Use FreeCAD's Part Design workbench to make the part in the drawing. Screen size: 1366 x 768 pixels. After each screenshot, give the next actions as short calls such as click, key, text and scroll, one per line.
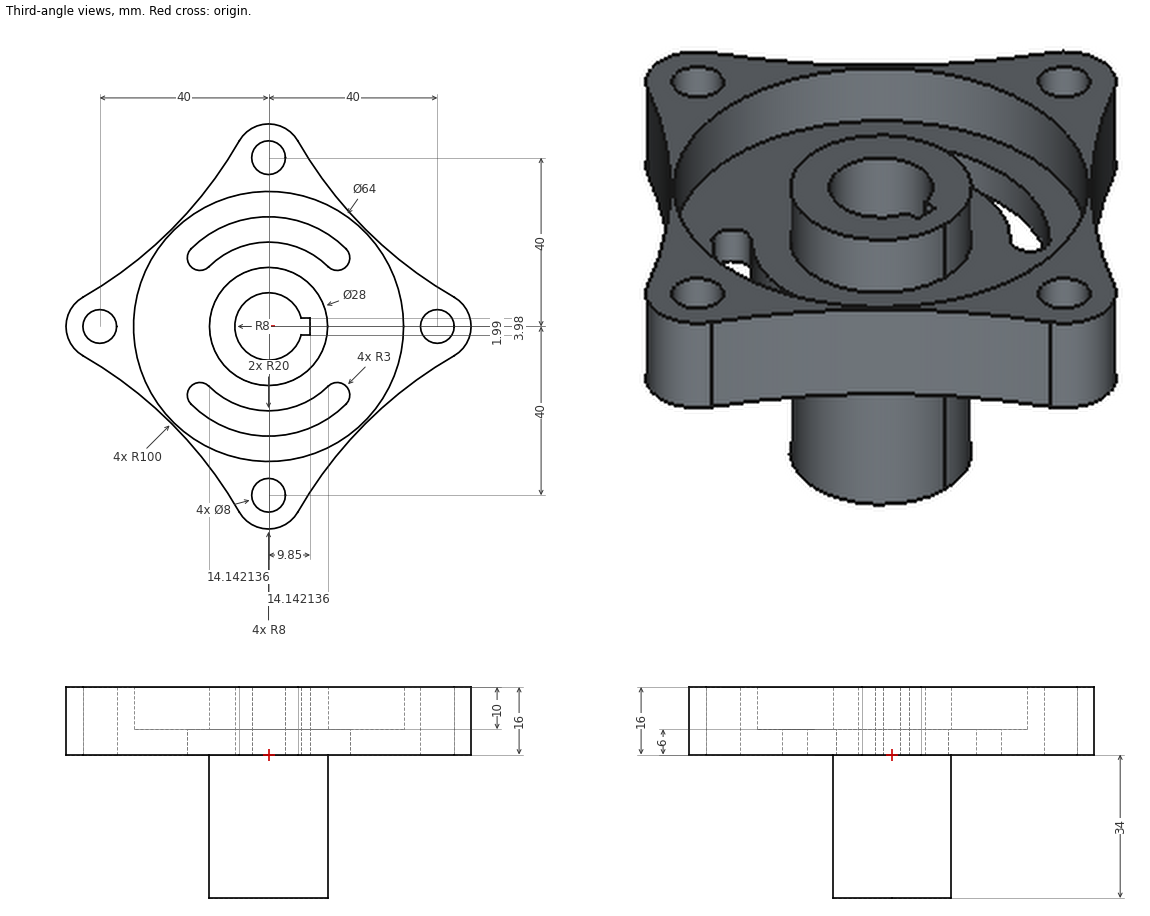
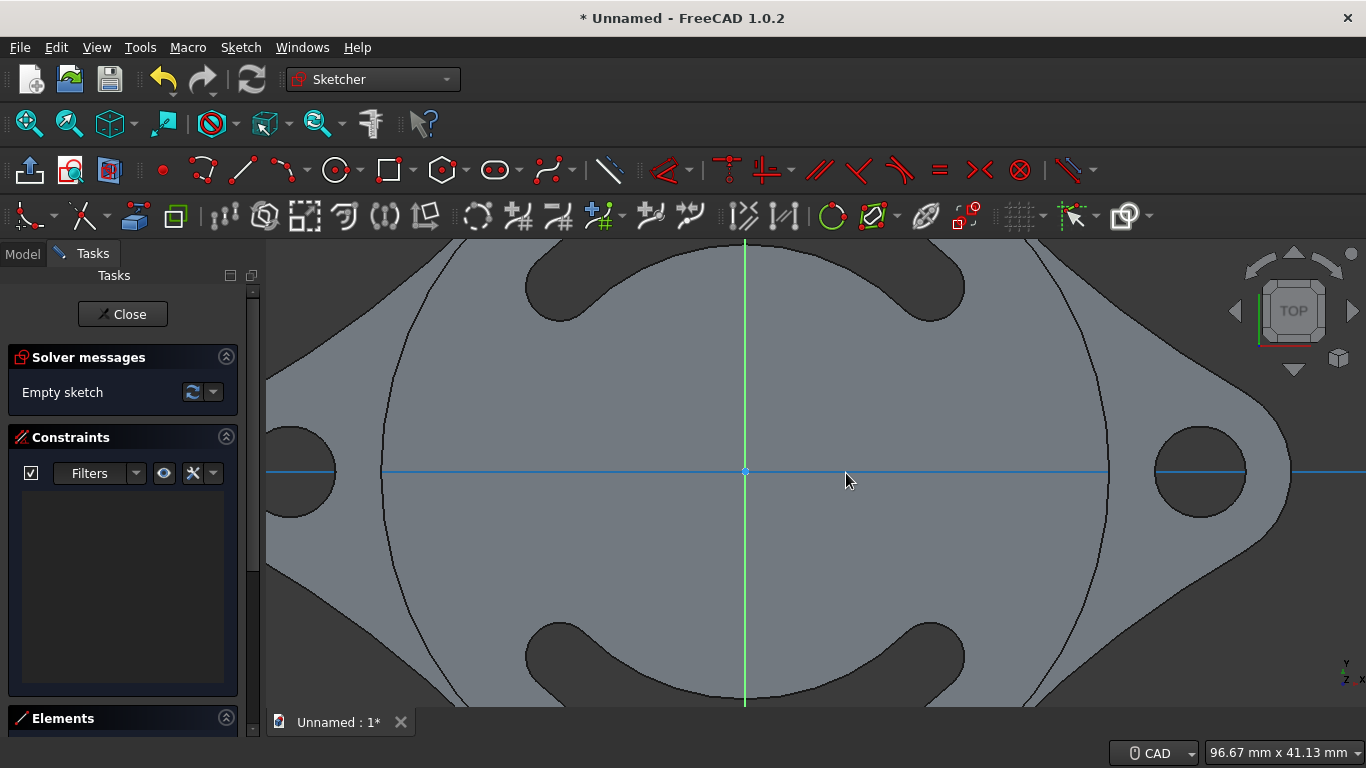
click(336, 170)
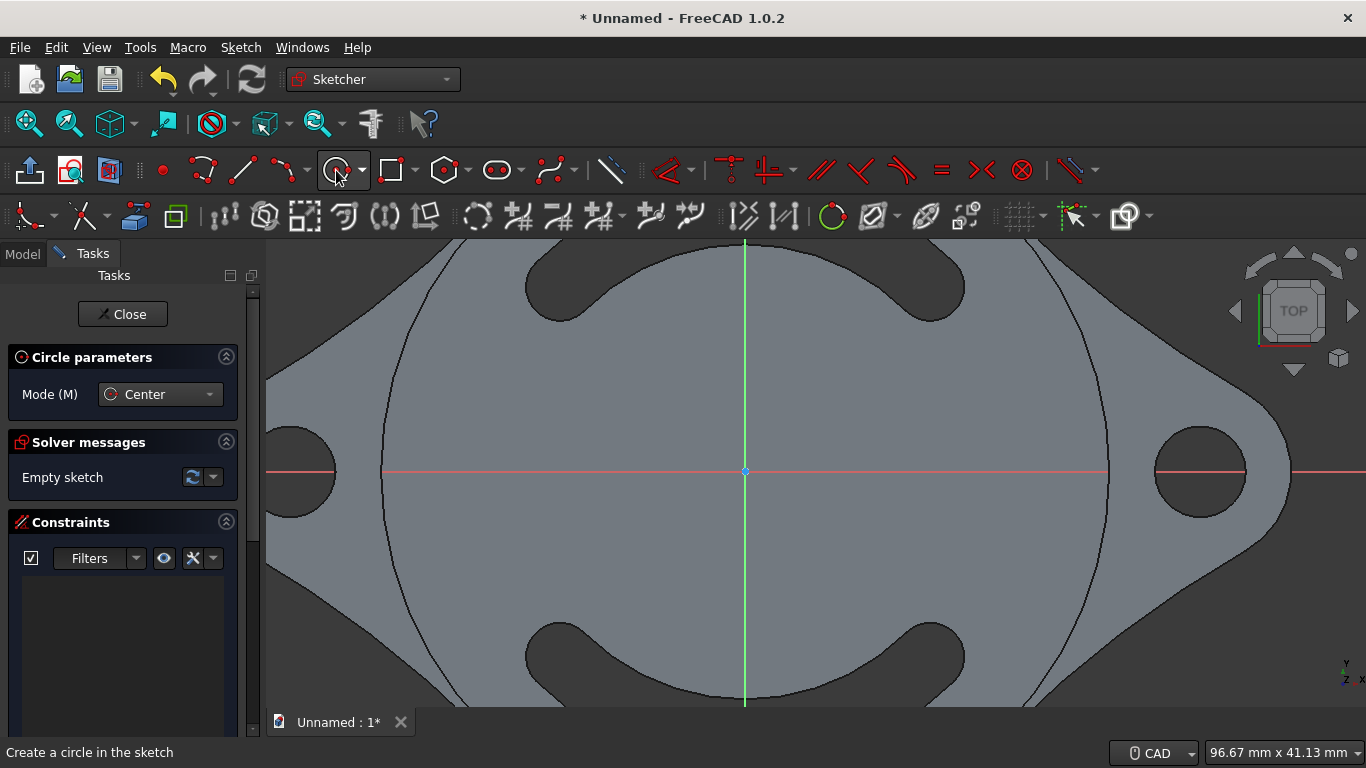
click(745, 472)
move(858, 359)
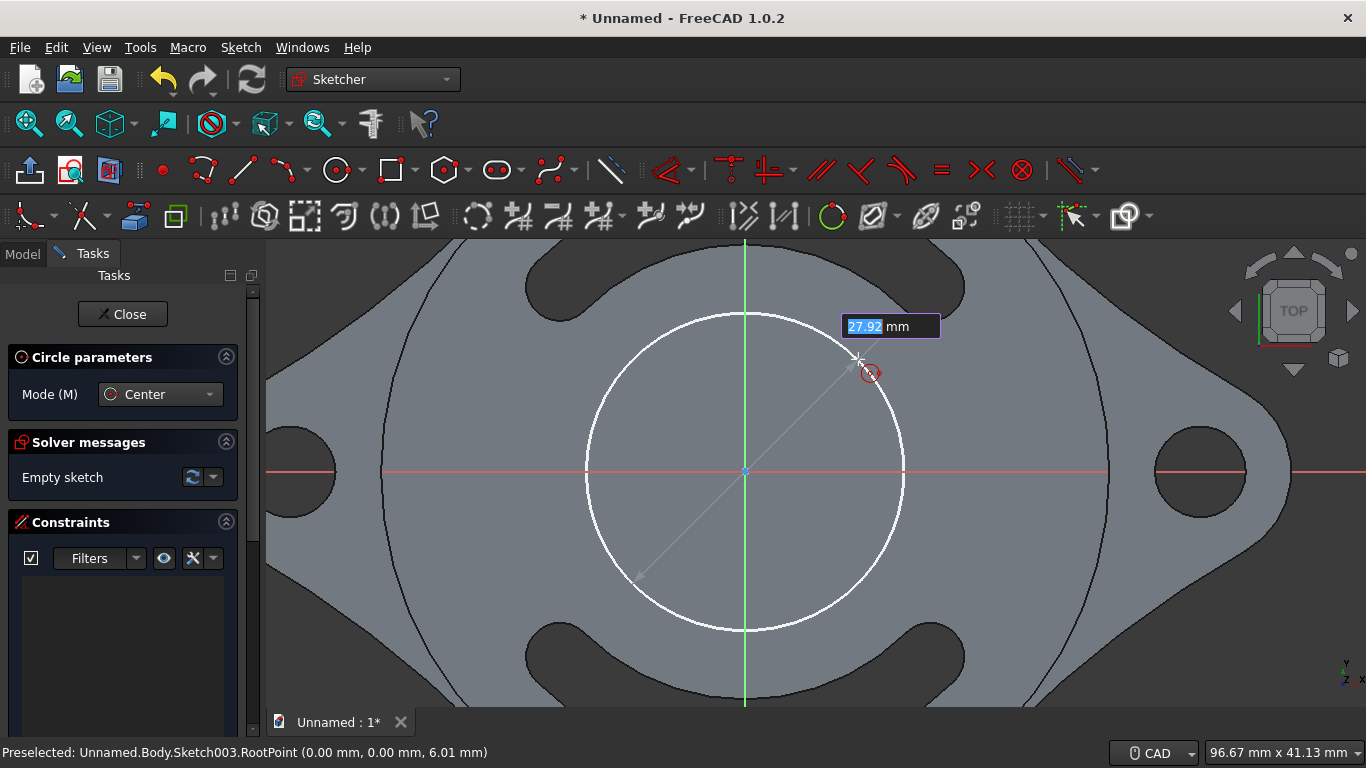
text(28)
key(Return)
key(Escape)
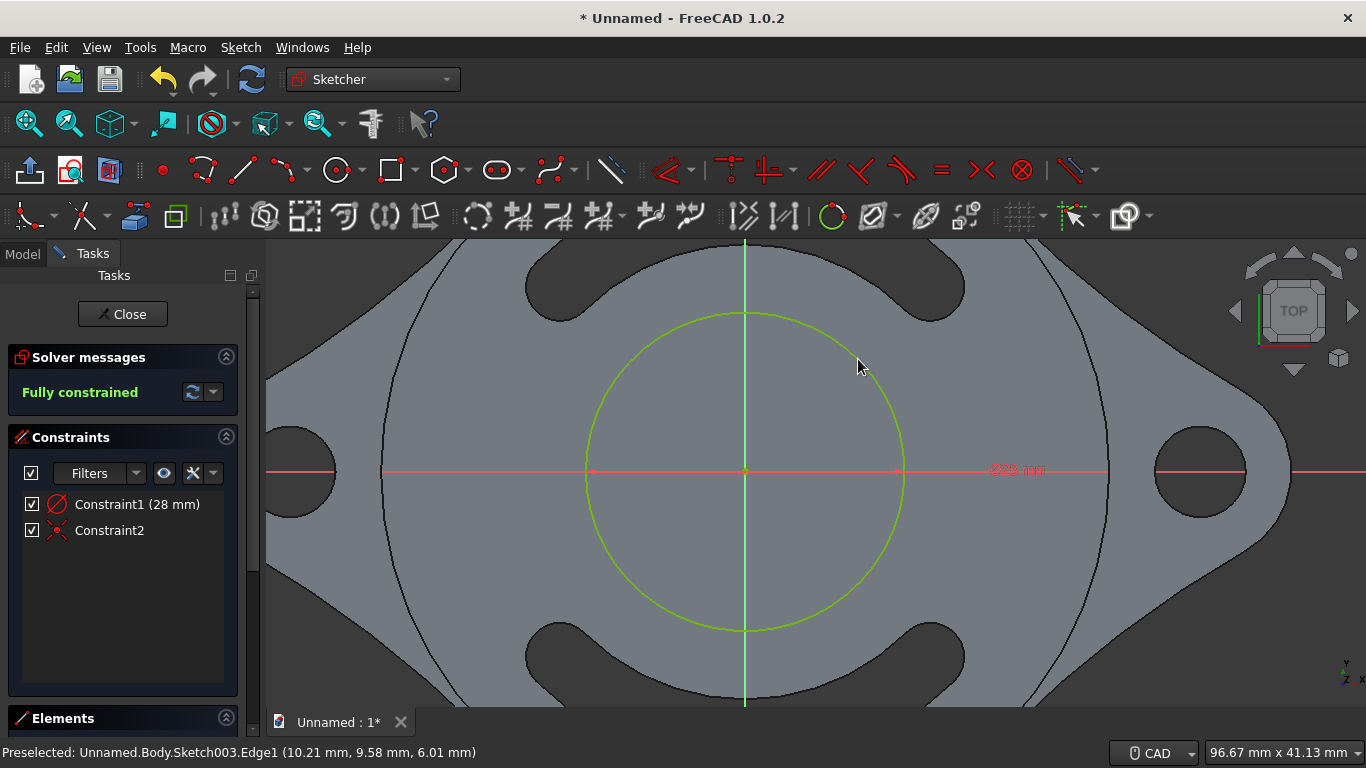
click(123, 314)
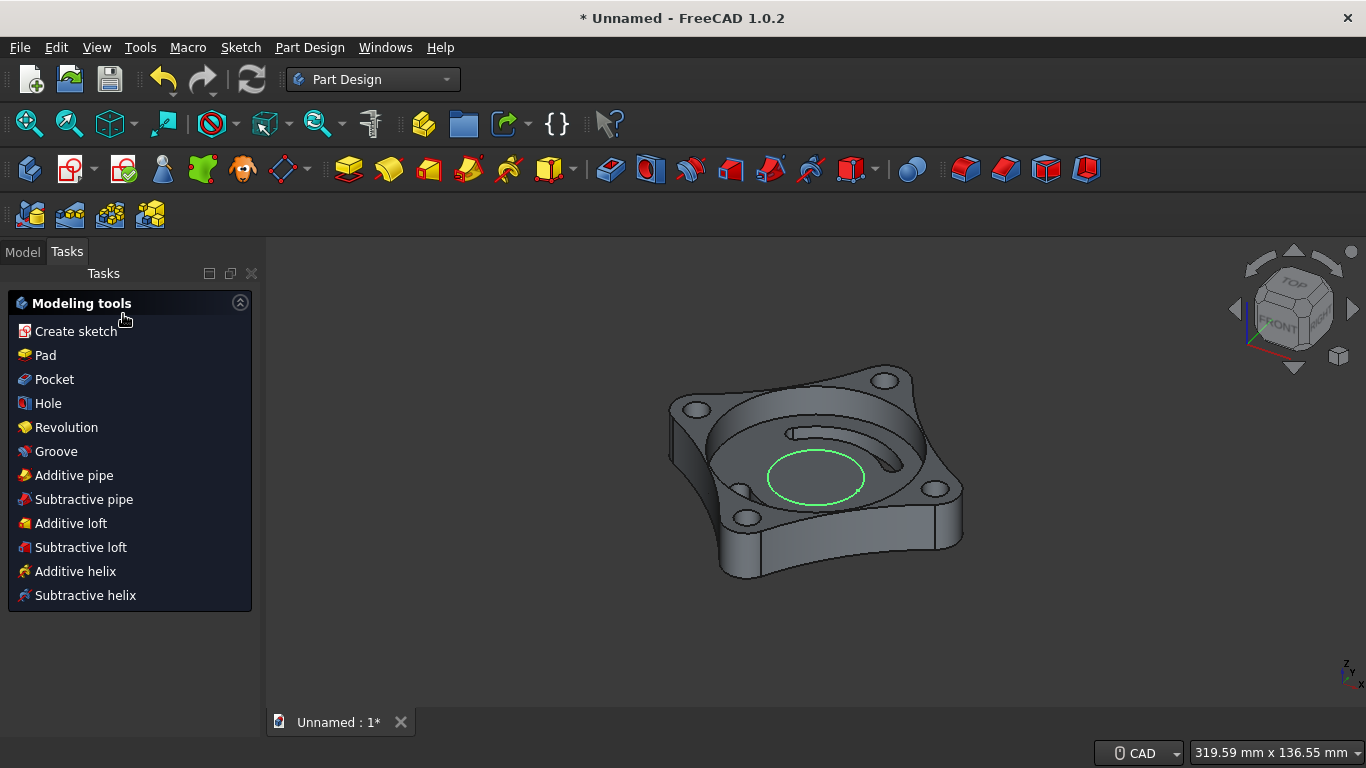
click(350, 170)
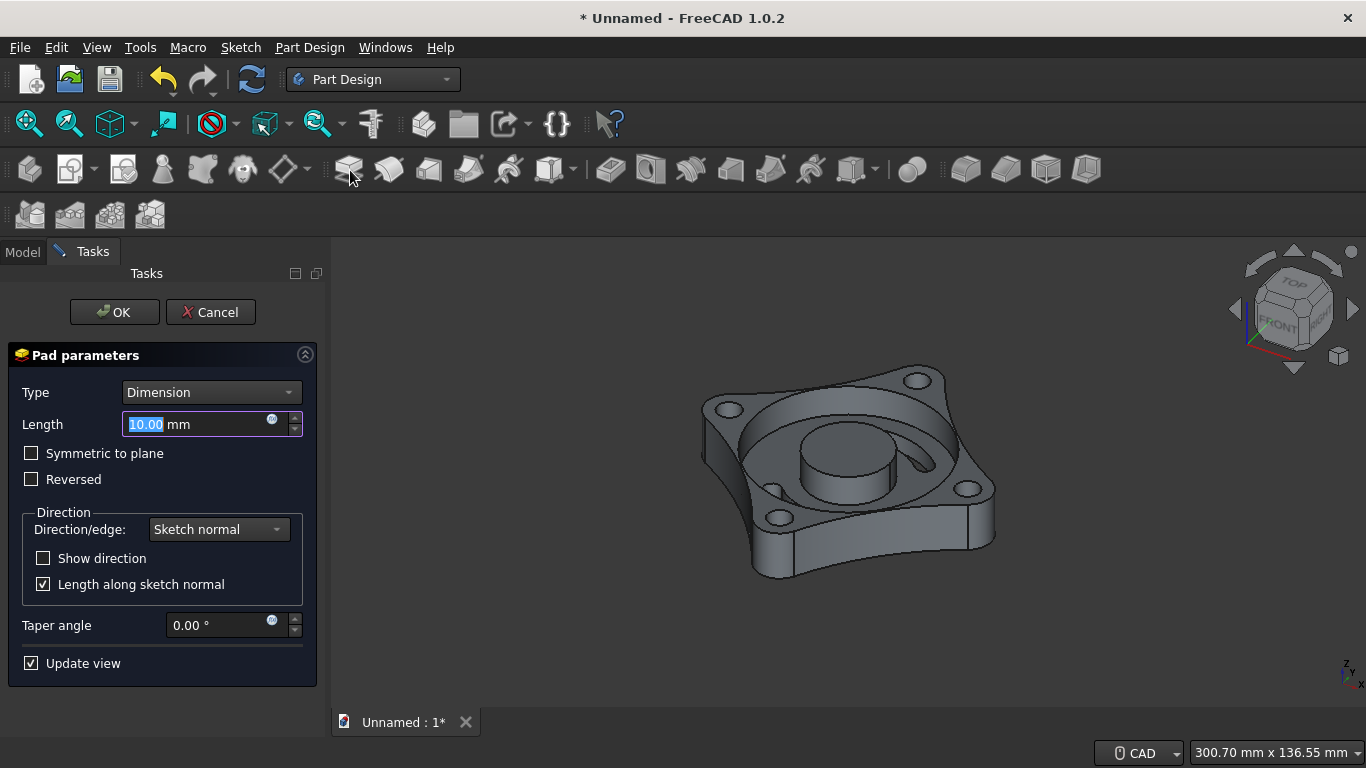
text(10)
key(Tab)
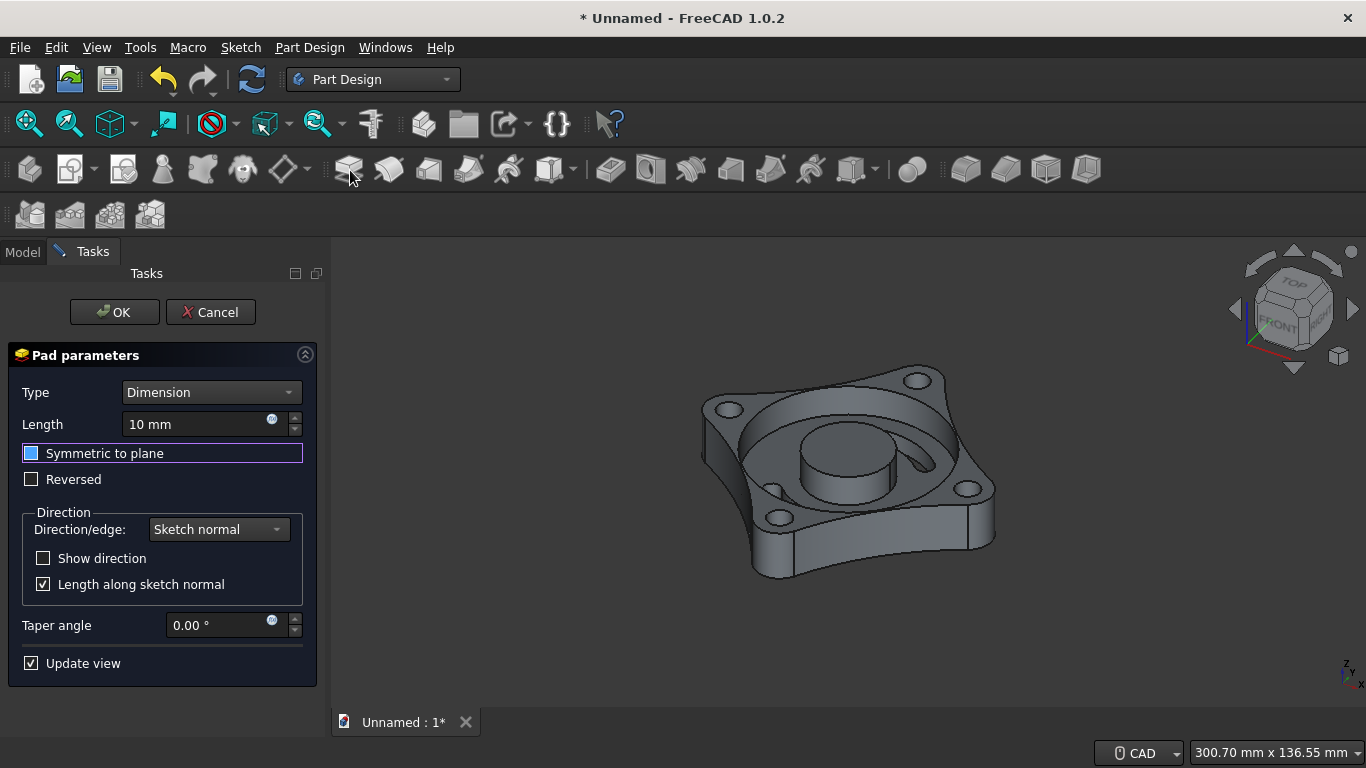
click(115, 312)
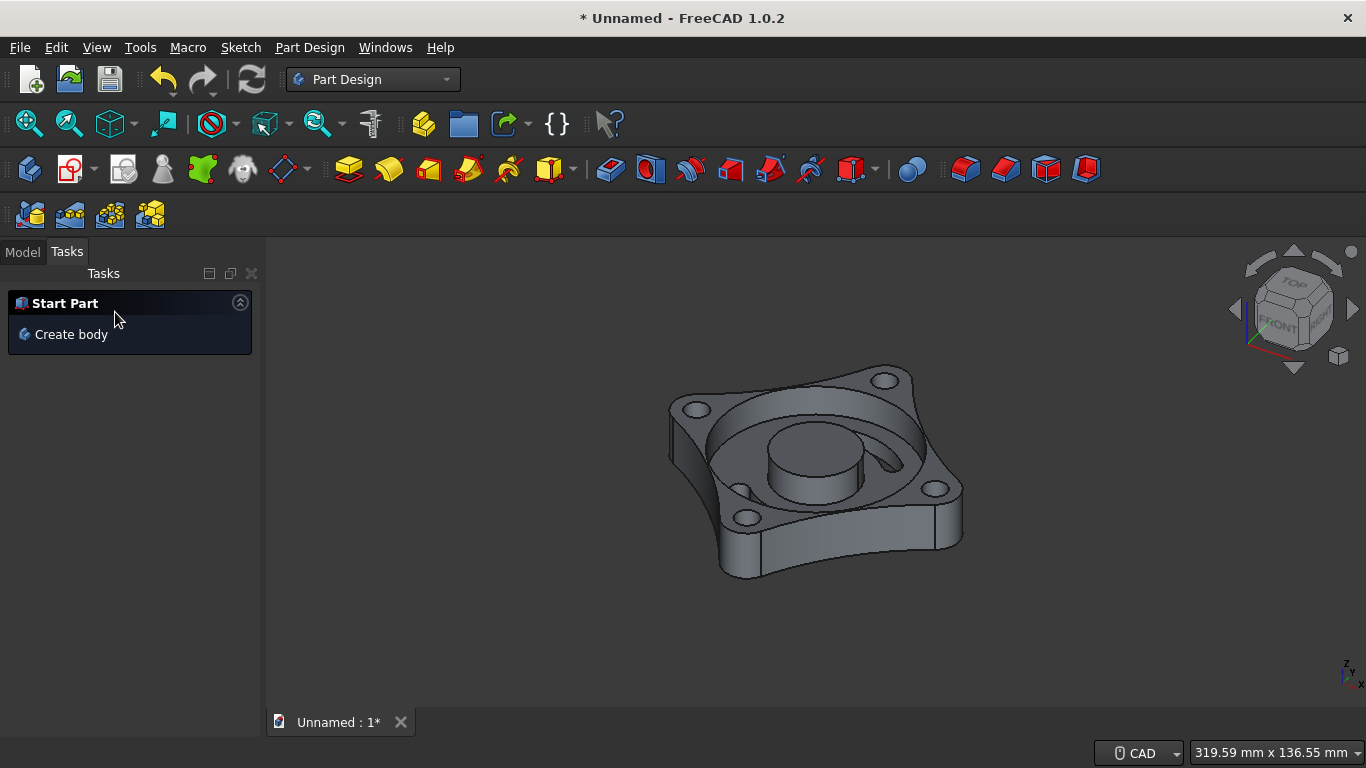
click(23, 251)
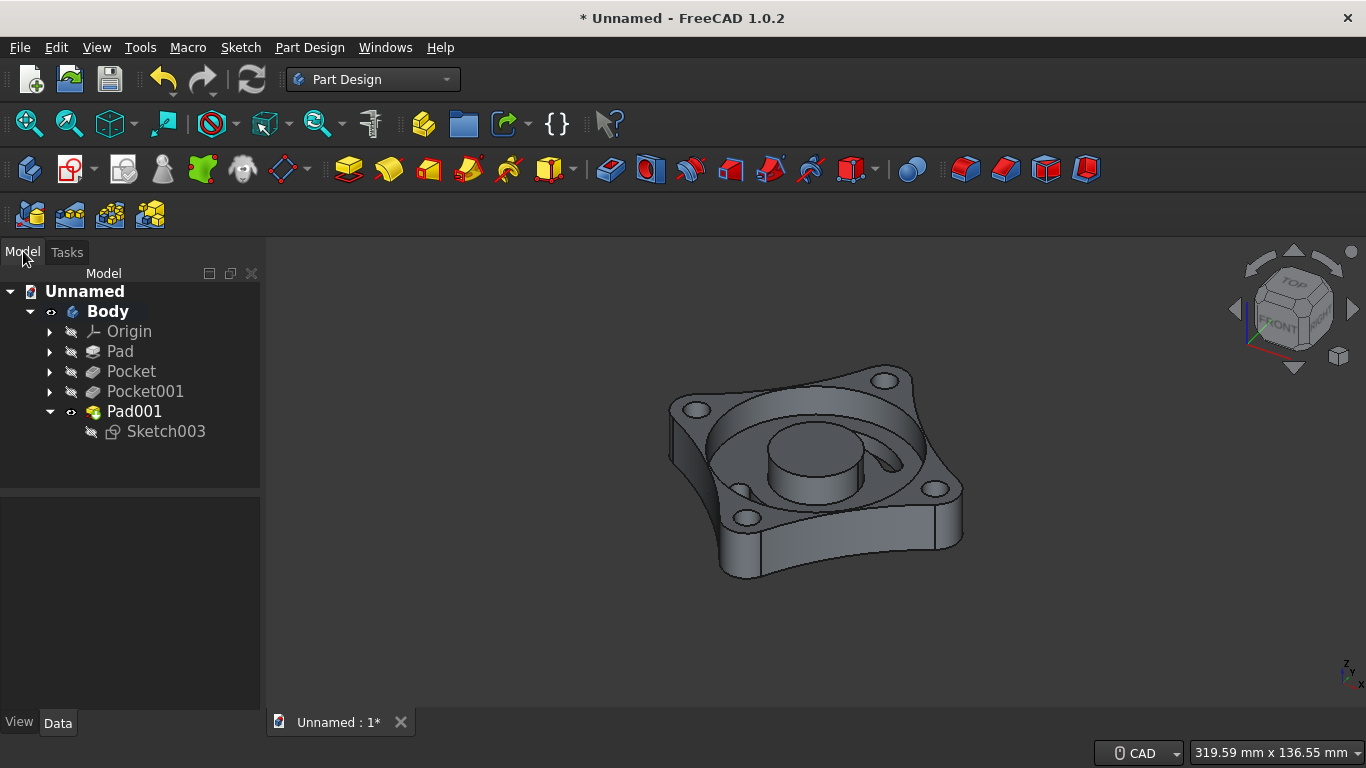
click(50, 332)